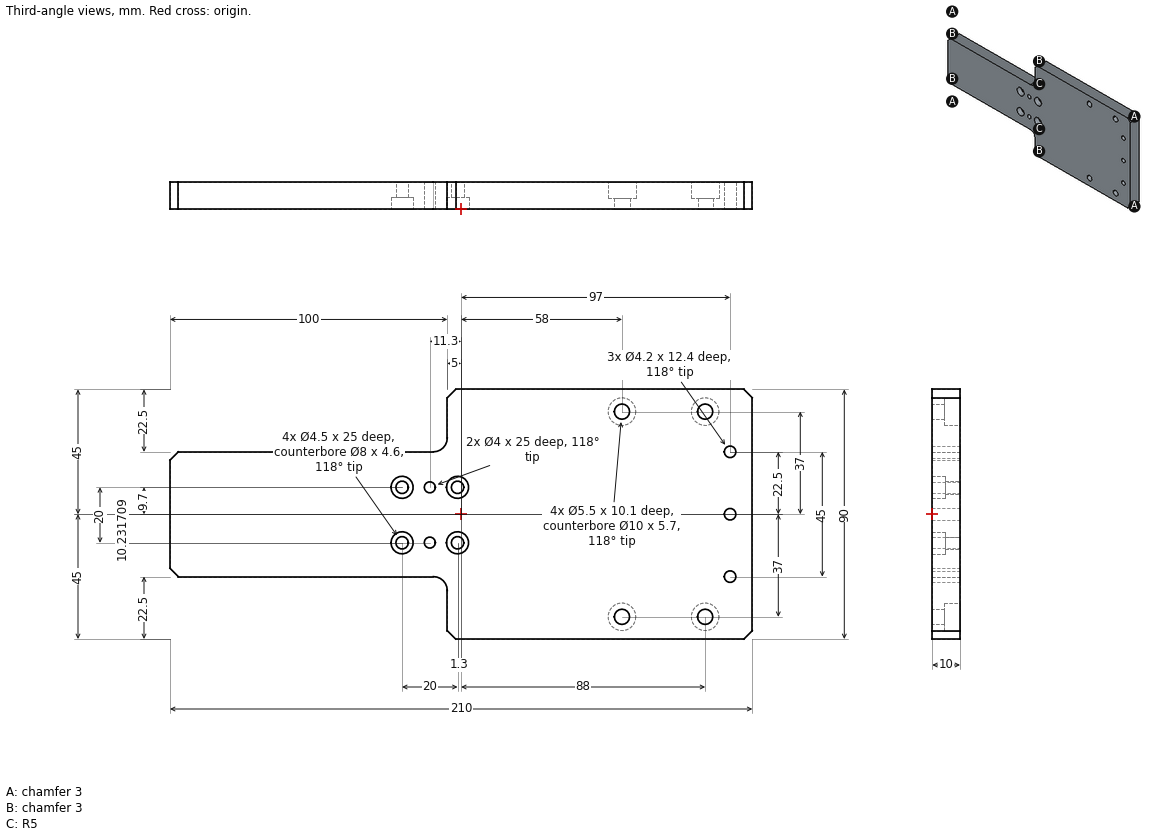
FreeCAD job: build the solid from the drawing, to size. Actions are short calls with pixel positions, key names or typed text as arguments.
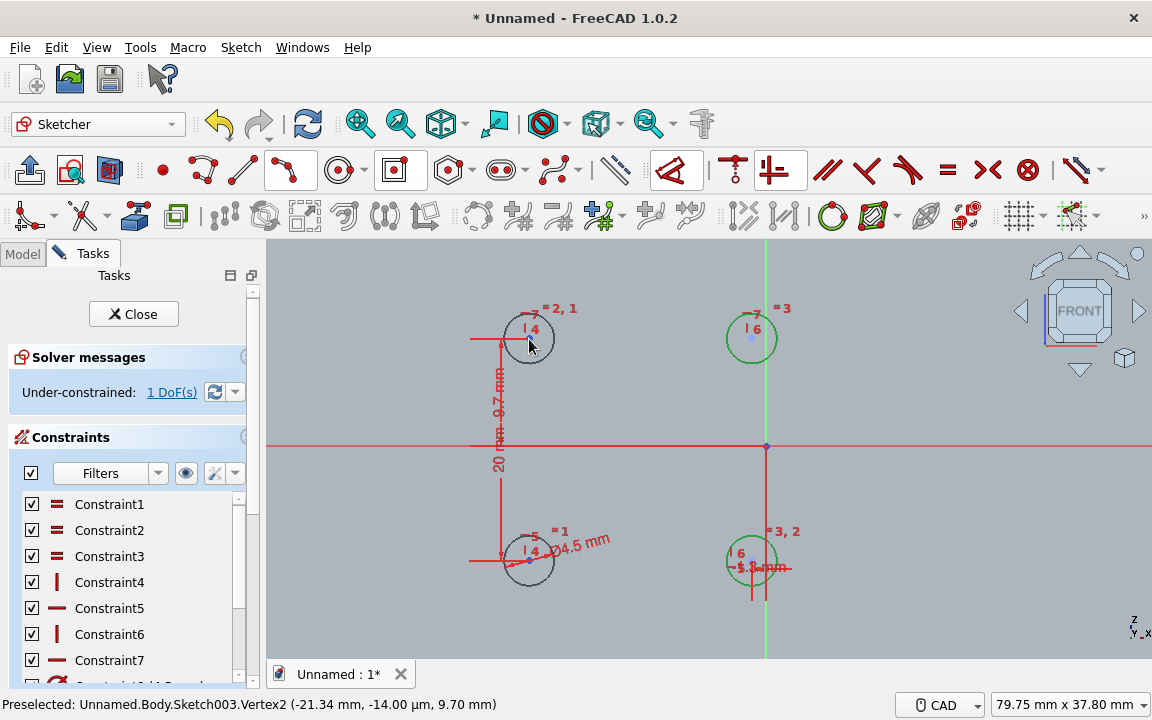
click(529, 561)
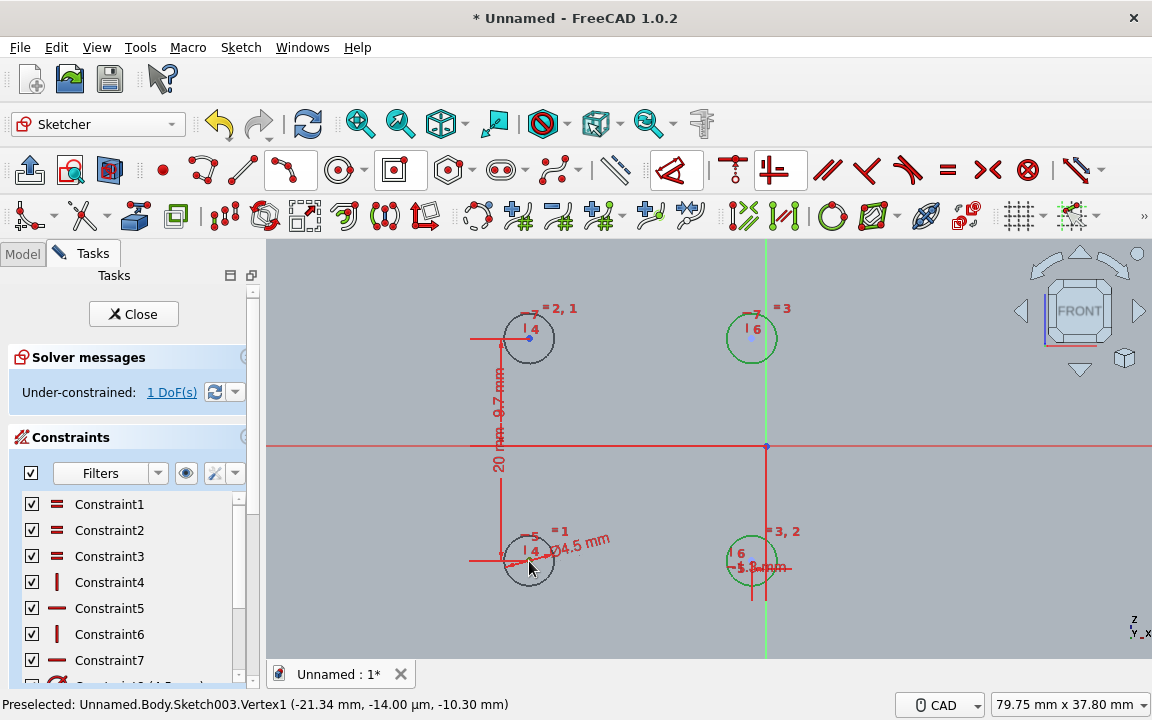
click(752, 561)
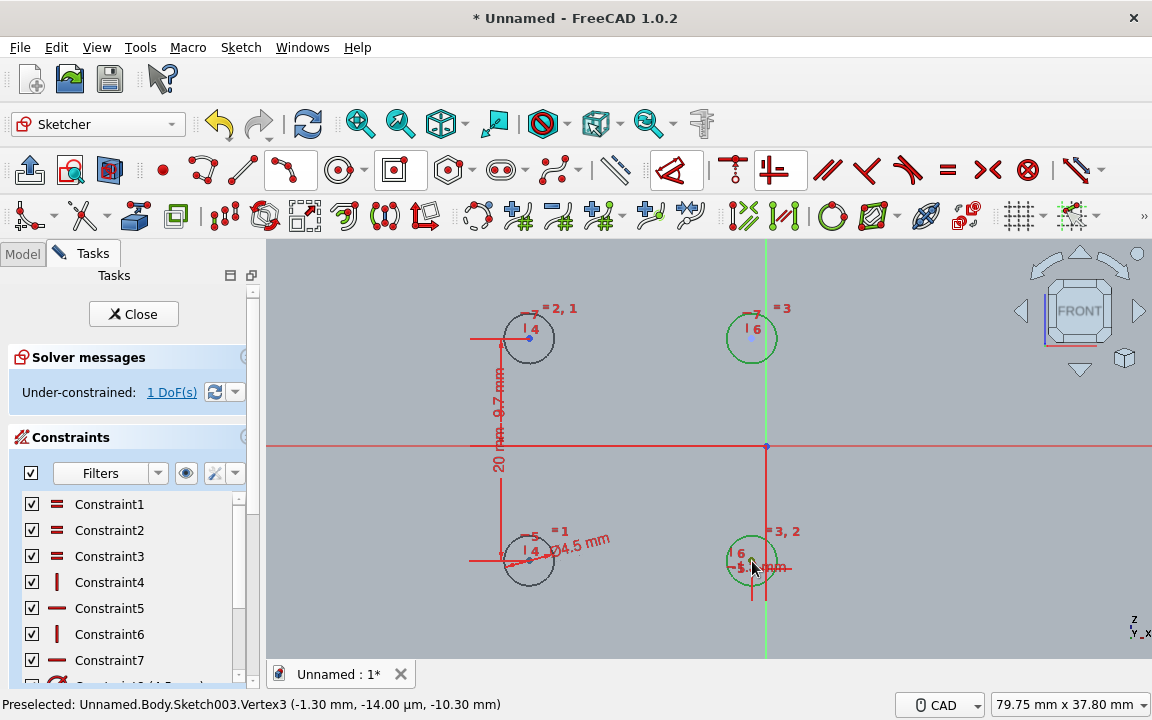
click(698, 170)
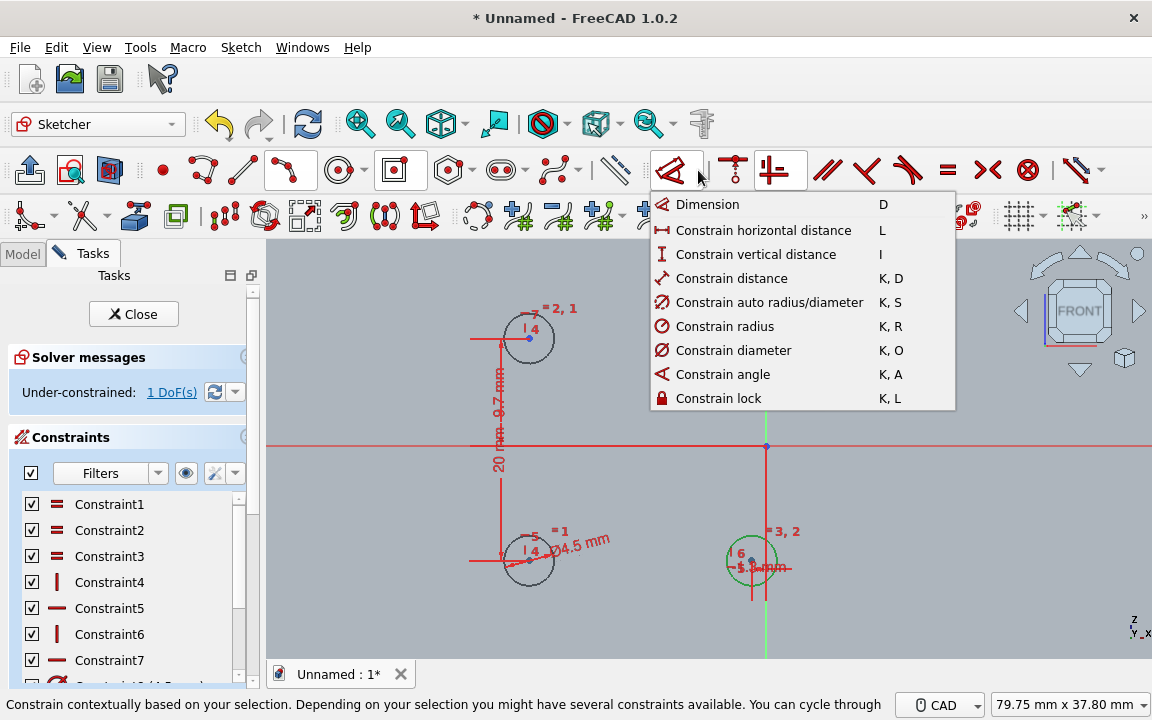
click(803, 230)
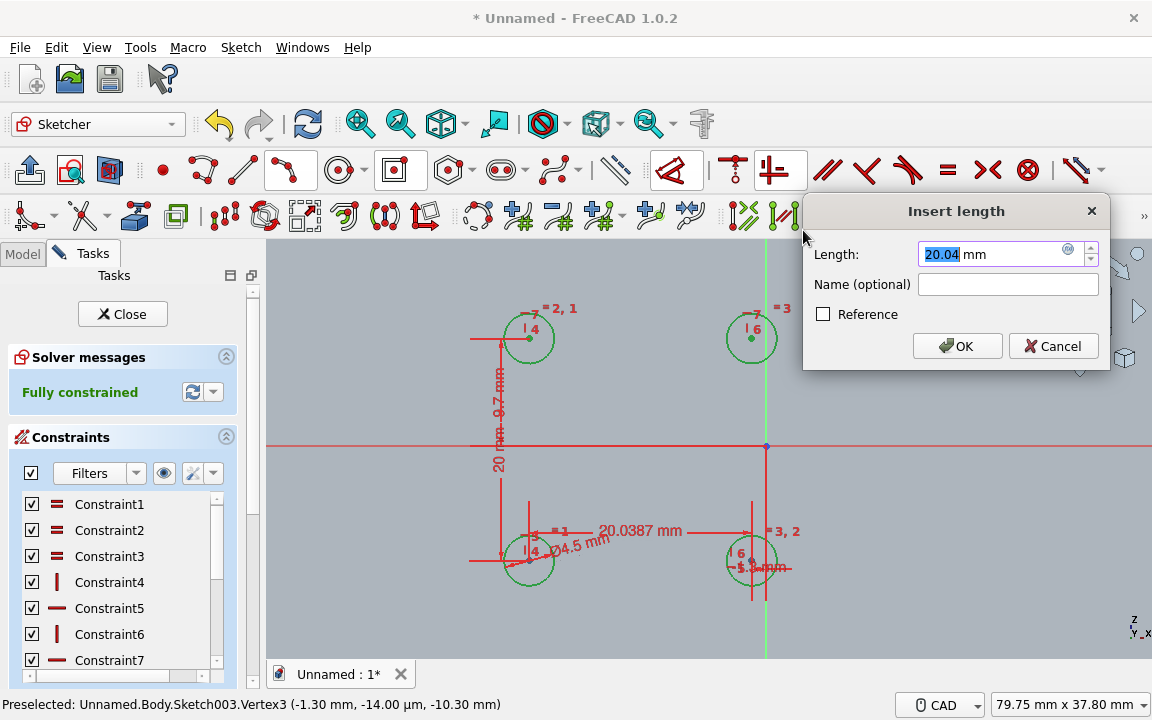
text(20)
key(Return)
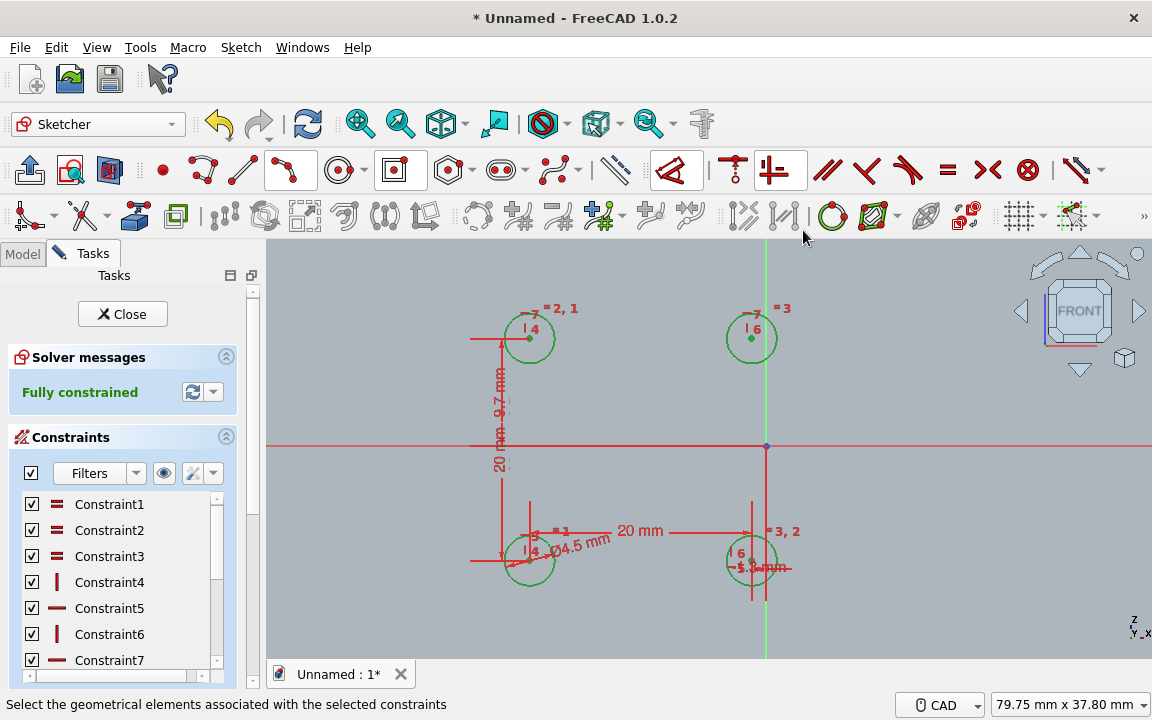
click(123, 314)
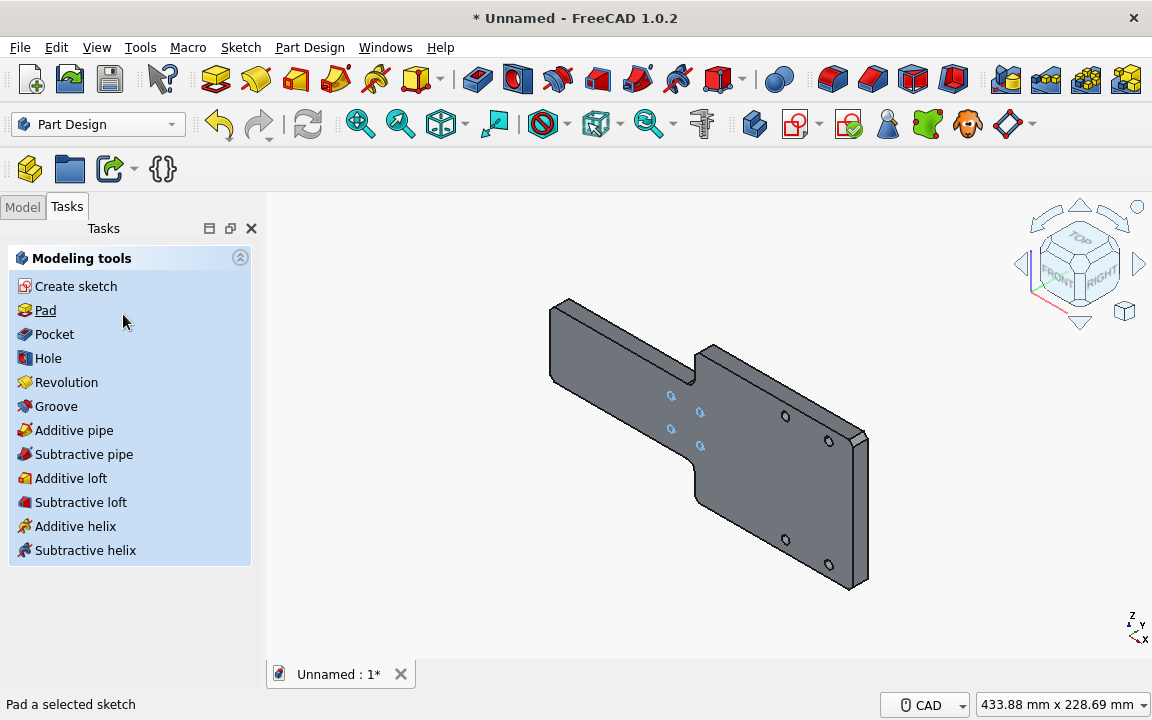
click(518, 80)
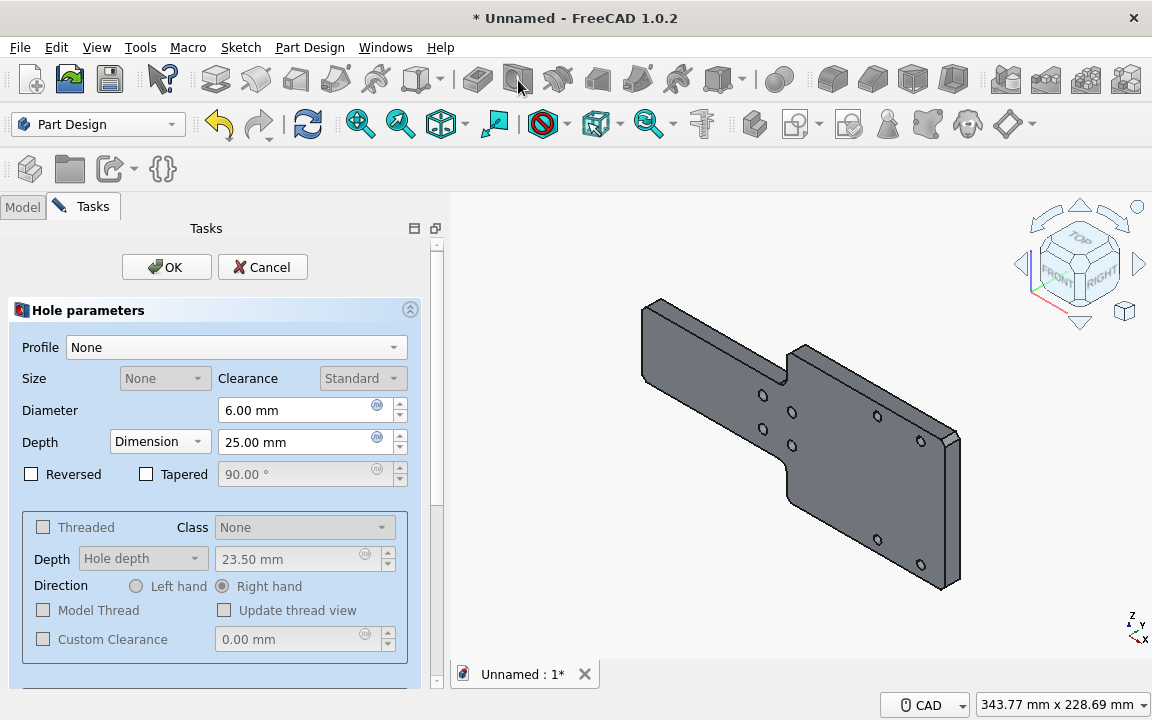
triple_click(305, 410)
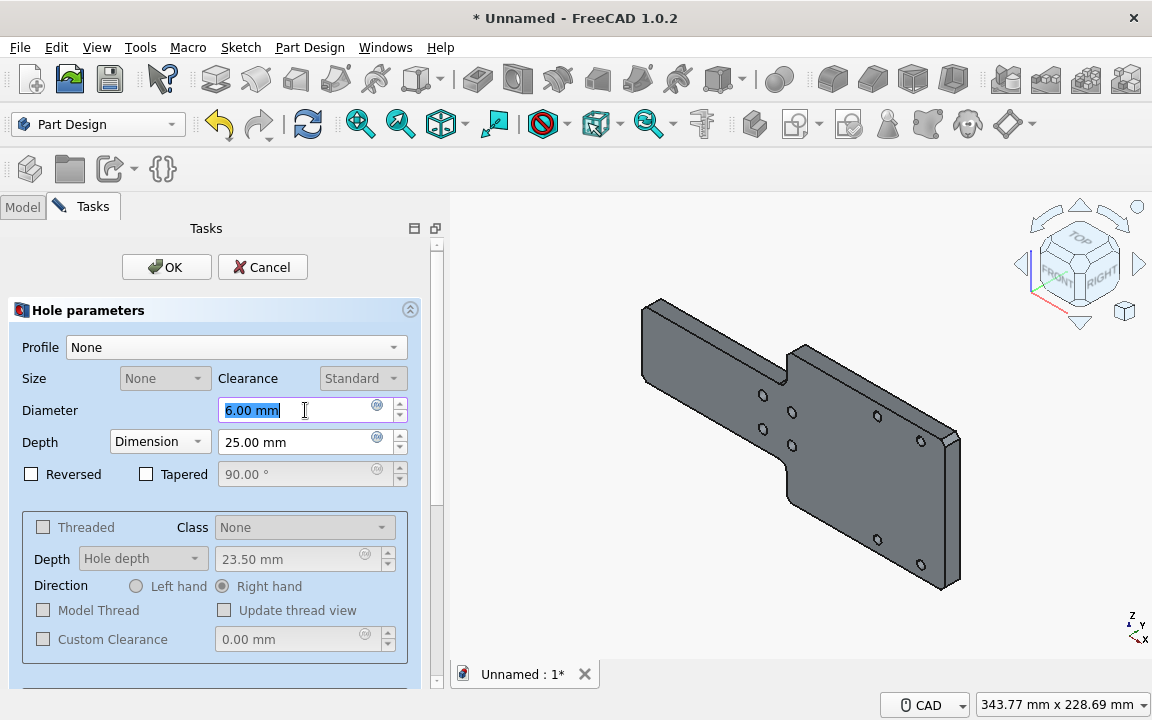
text(4.5)
key(Tab)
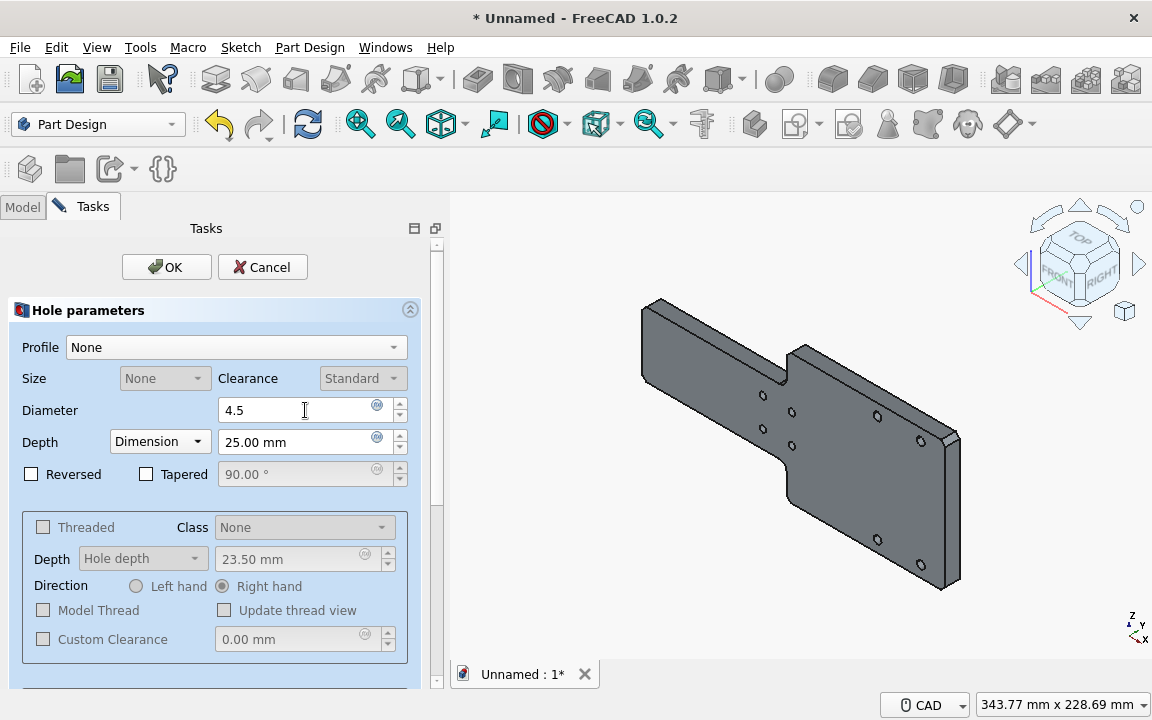
triple_click(305, 442)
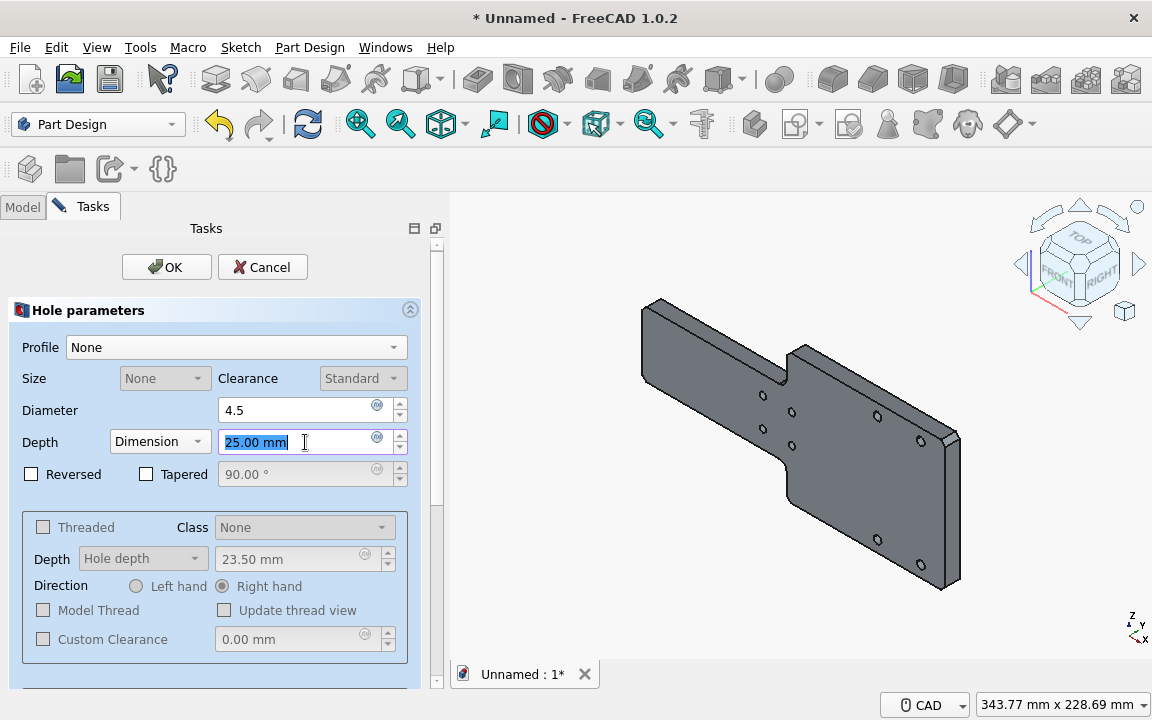
text(25)
key(Tab)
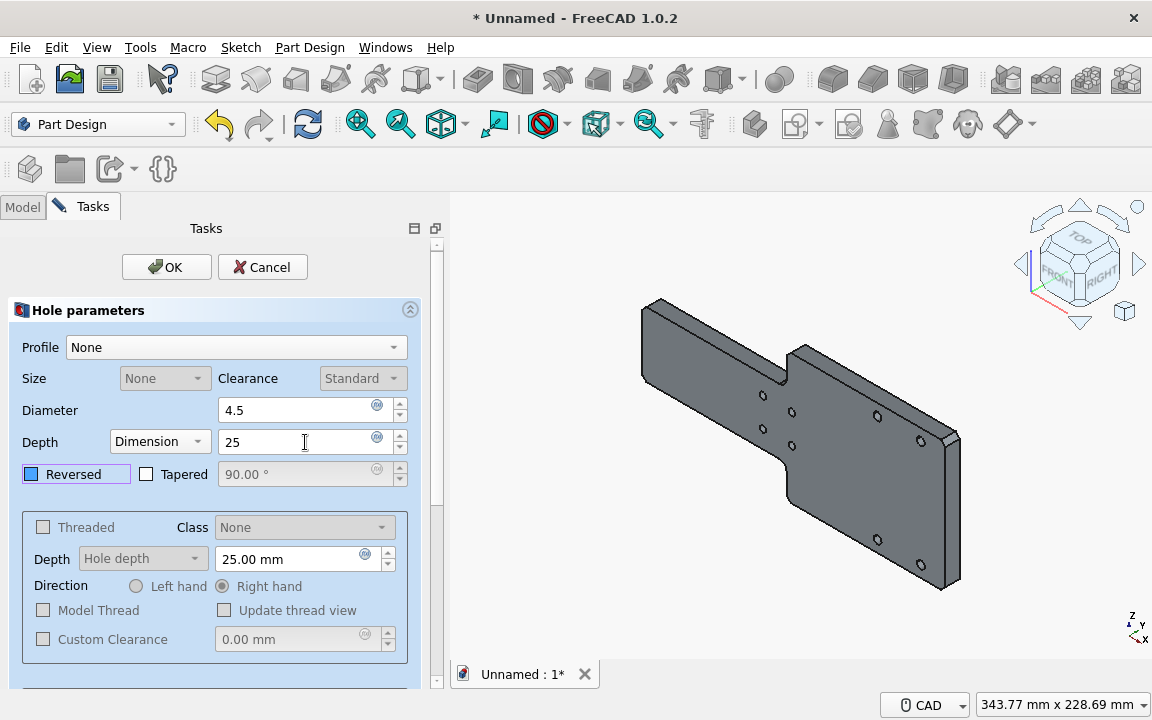
scroll(437, 463, down, 2)